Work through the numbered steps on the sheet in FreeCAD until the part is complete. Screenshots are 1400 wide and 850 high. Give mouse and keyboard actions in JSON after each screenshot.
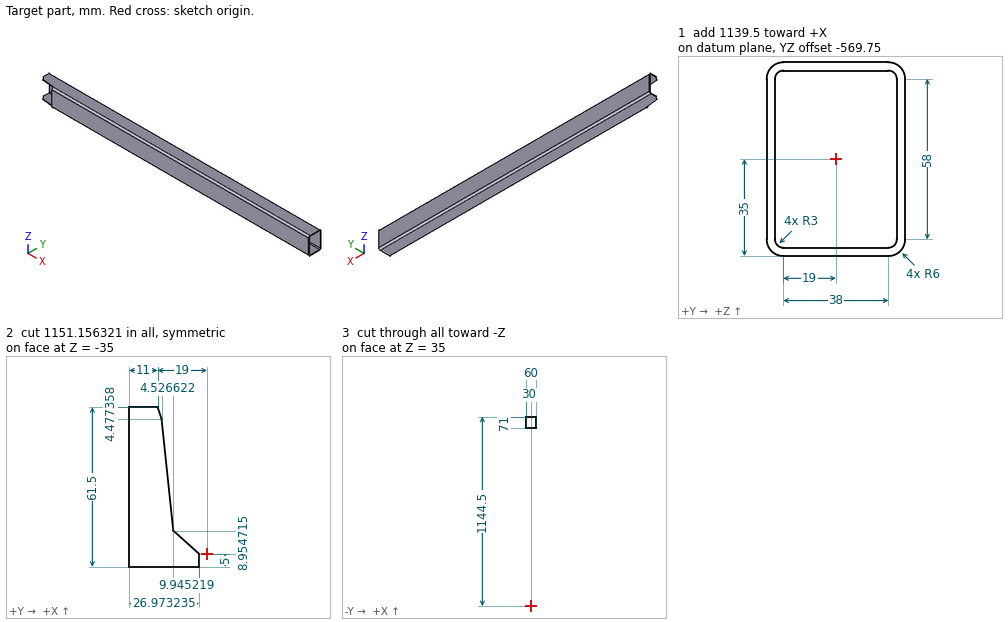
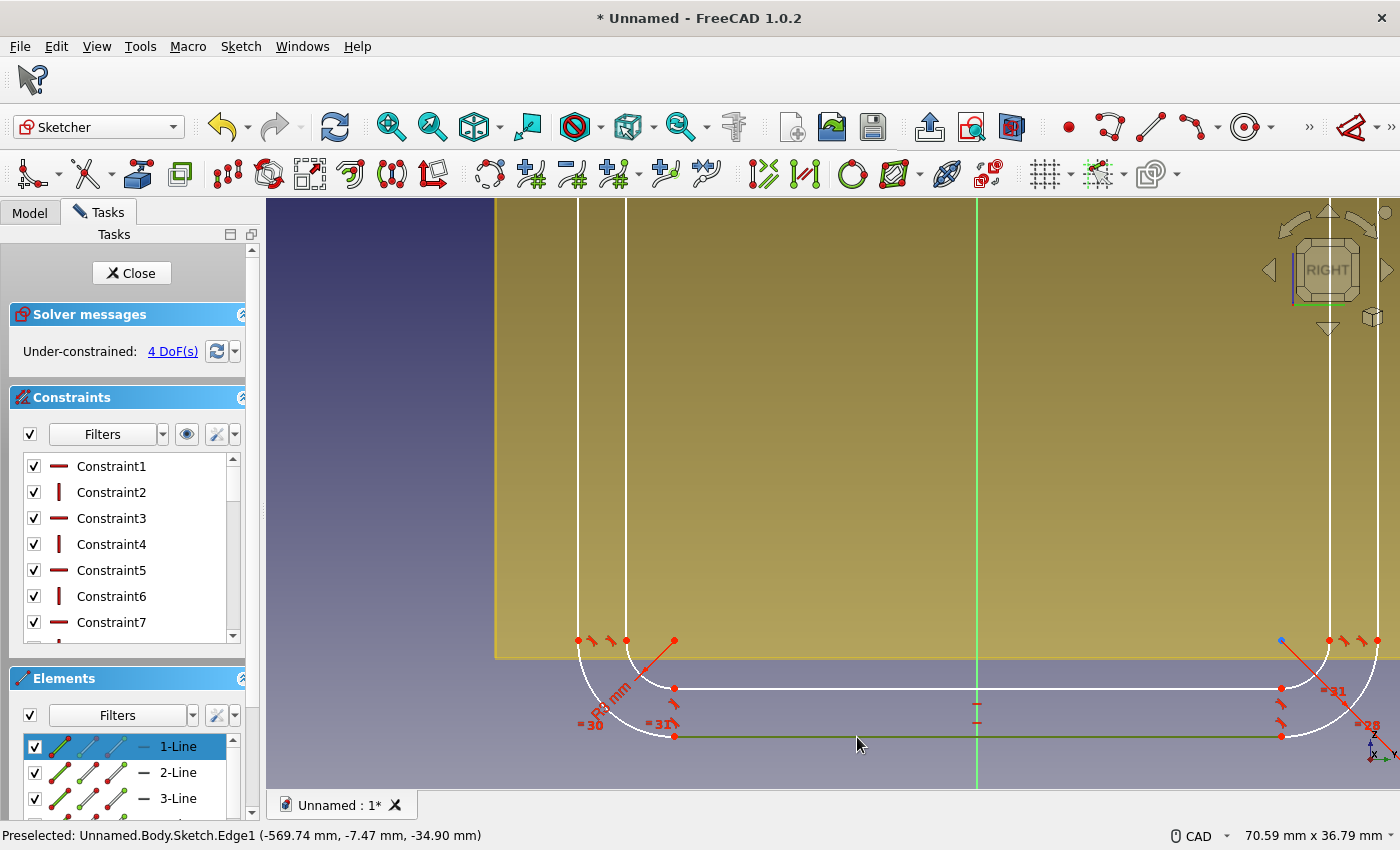
{"action": "key", "text": "l"}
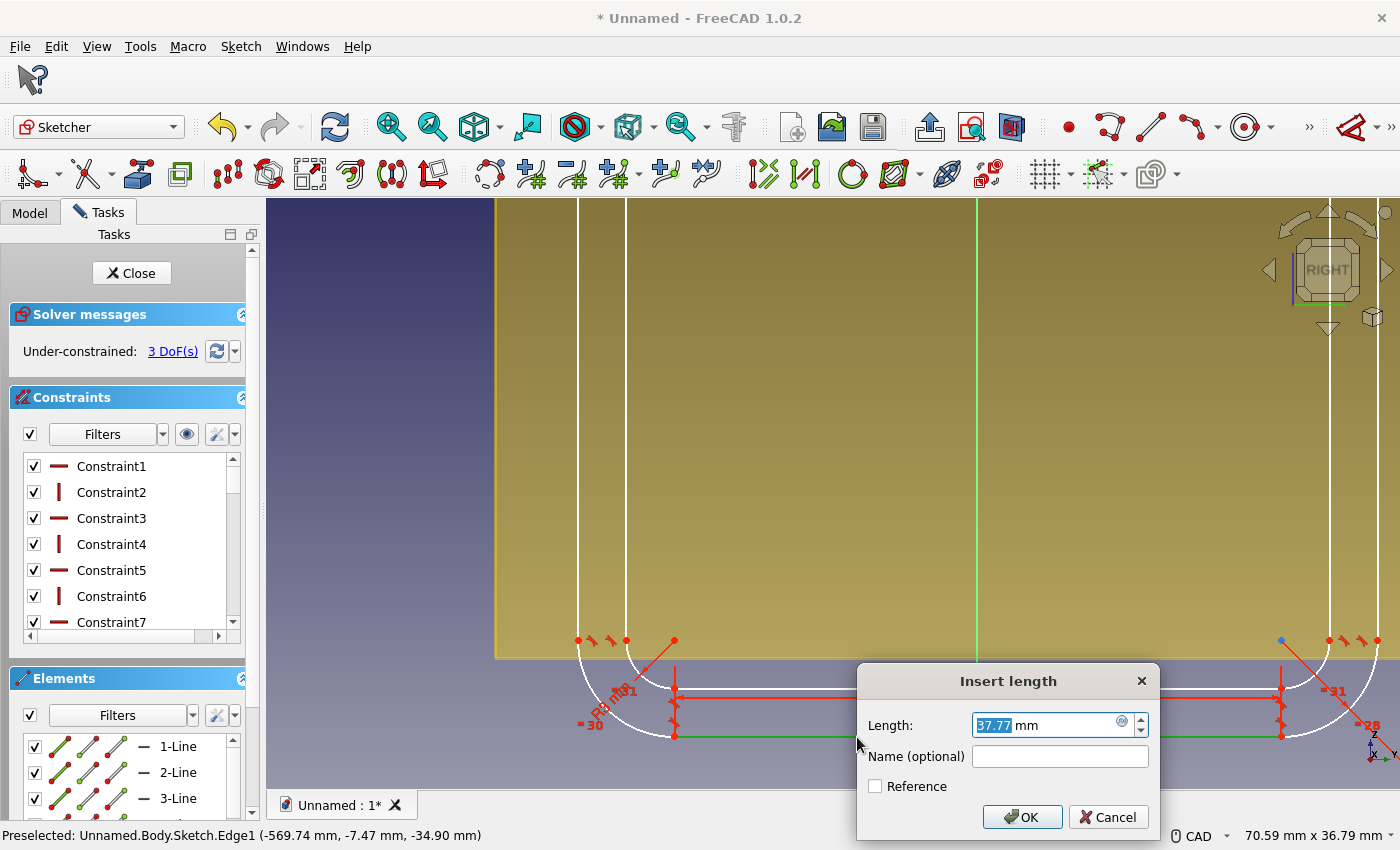
{"action": "type", "text": "38"}
{"action": "key", "text": "Return"}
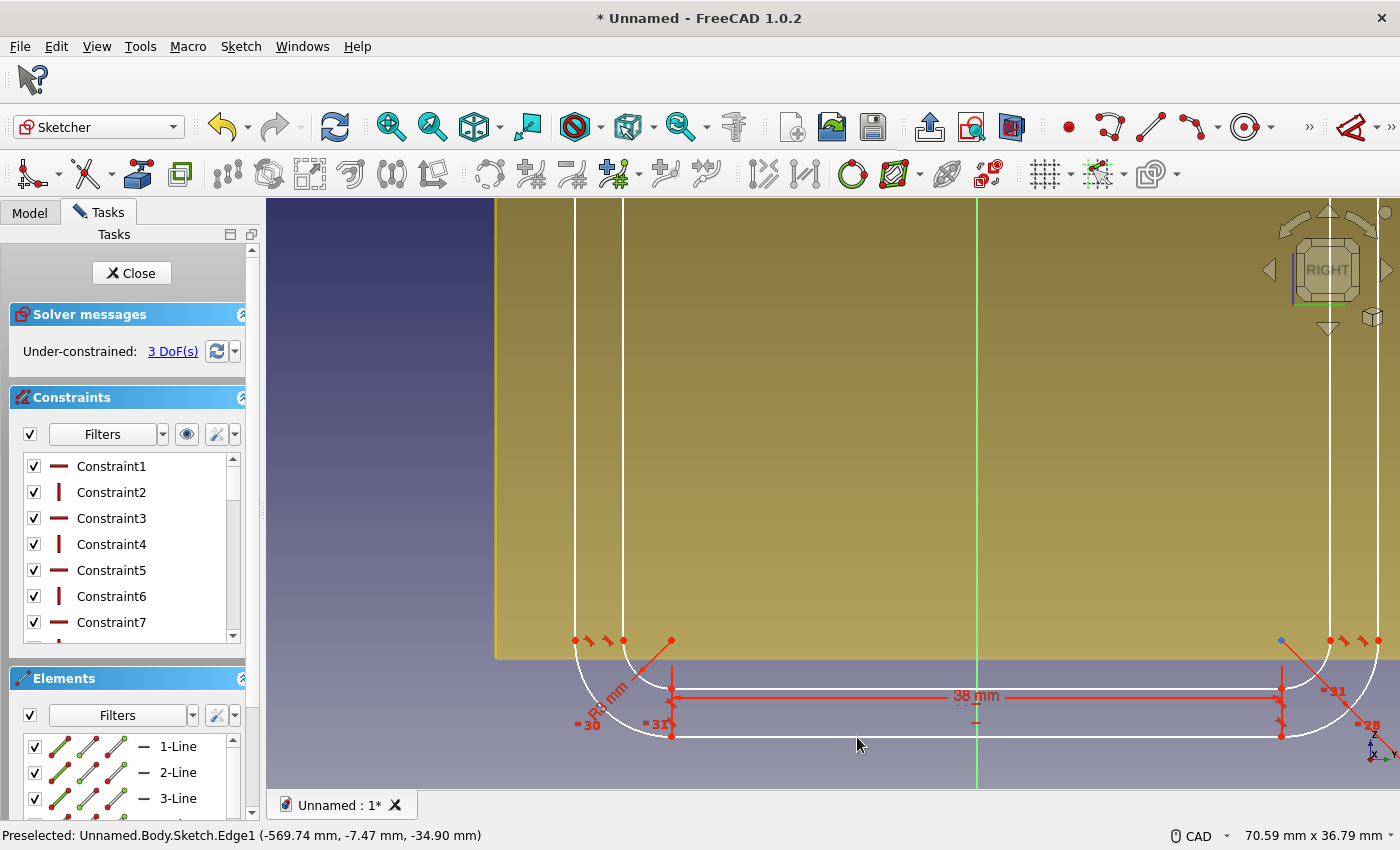
{"action": "scroll", "coordinate": [641, 678], "scroll_direction": "down", "scroll_amount": 5}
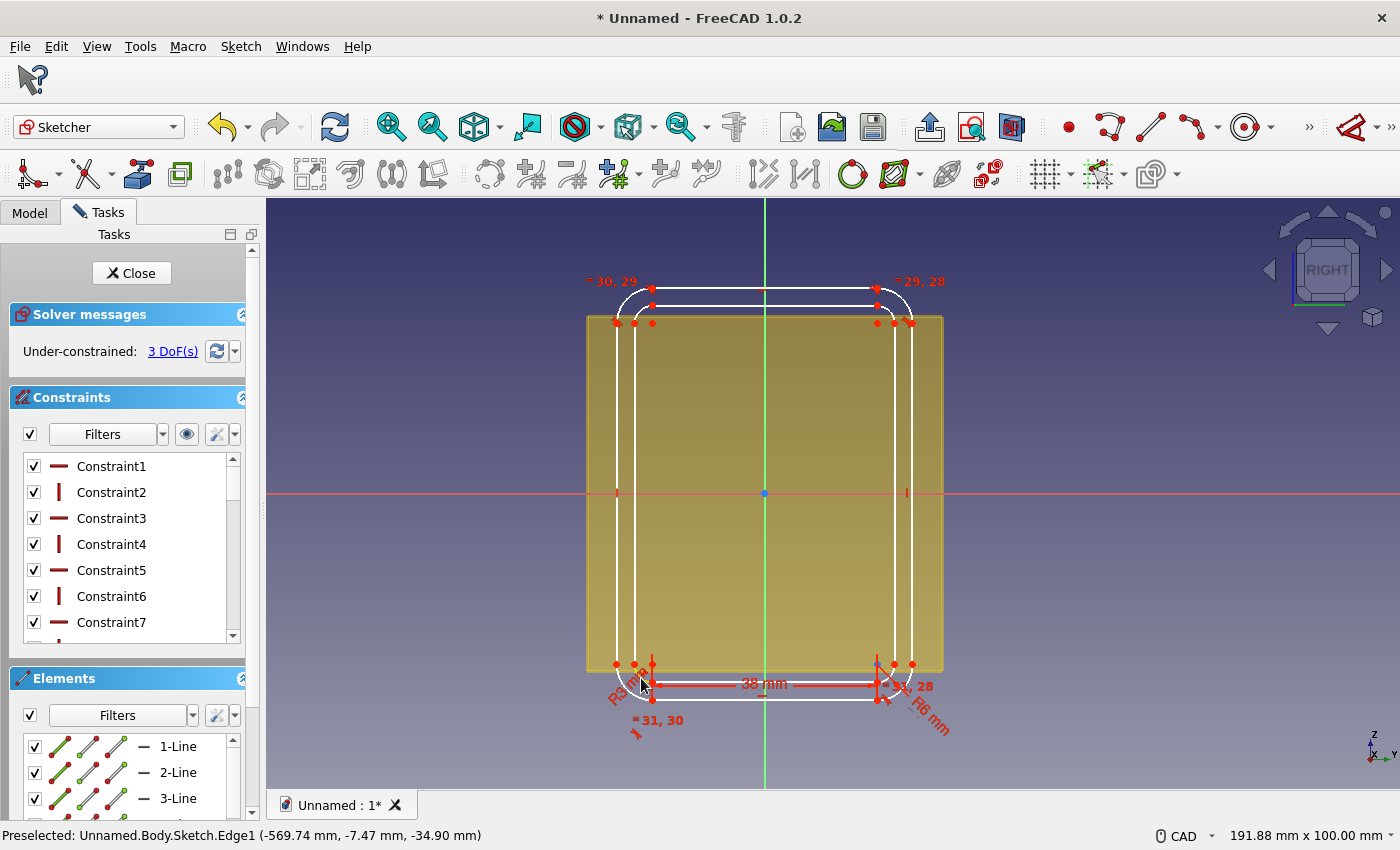
{"action": "left_click", "coordinate": [912, 562]}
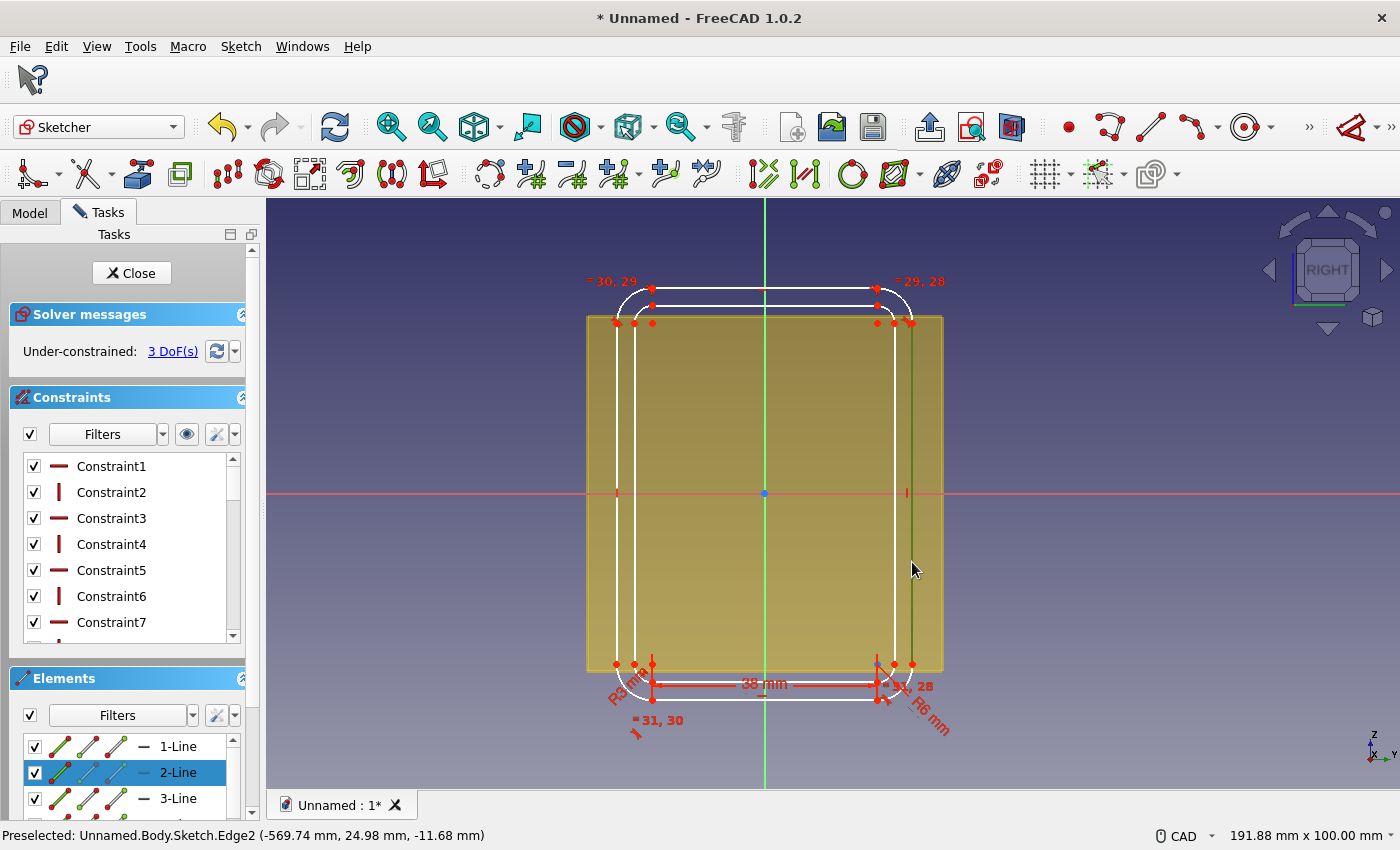
{"action": "key", "text": "i"}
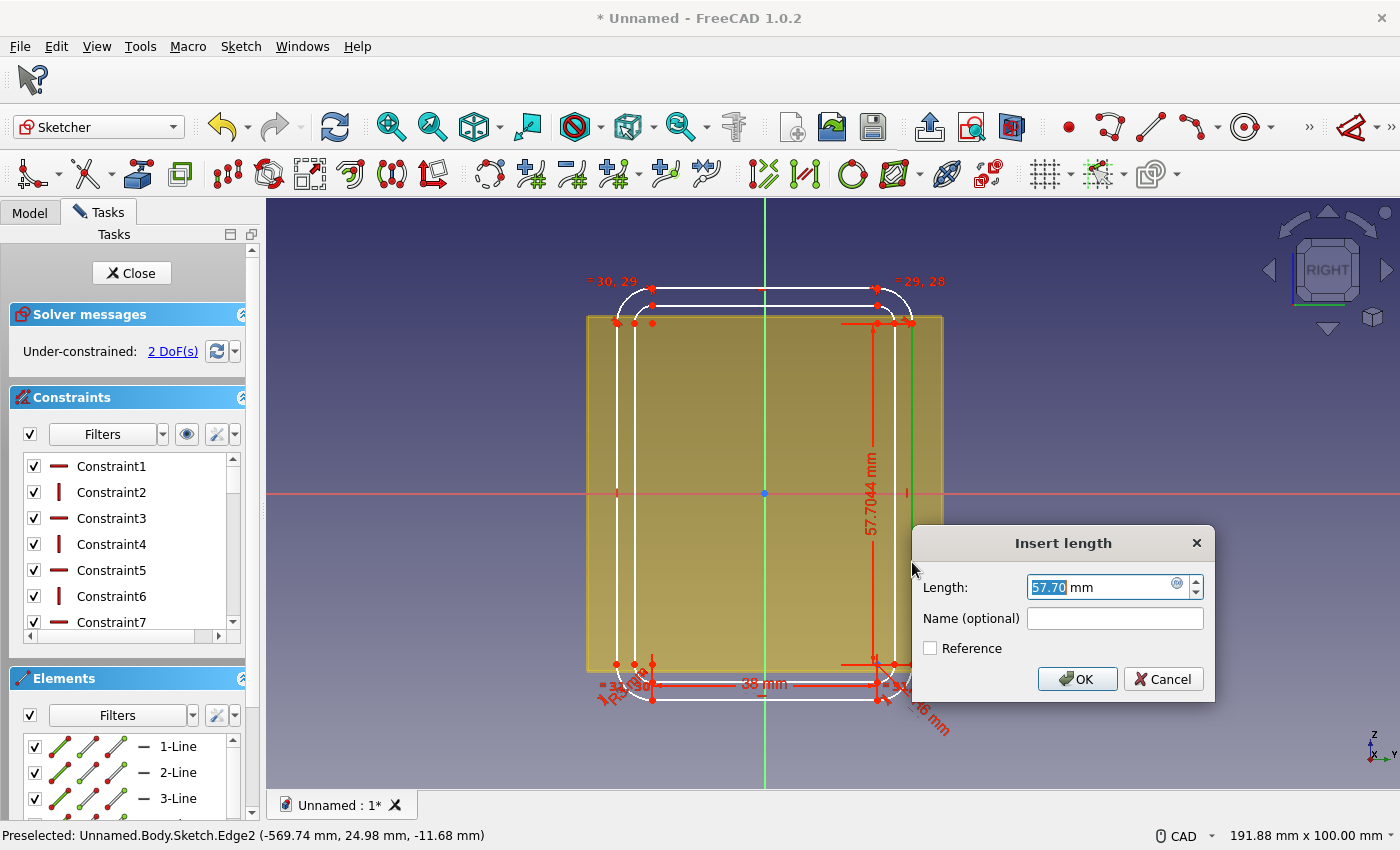
{"action": "type", "text": "58"}
{"action": "key", "text": "Return"}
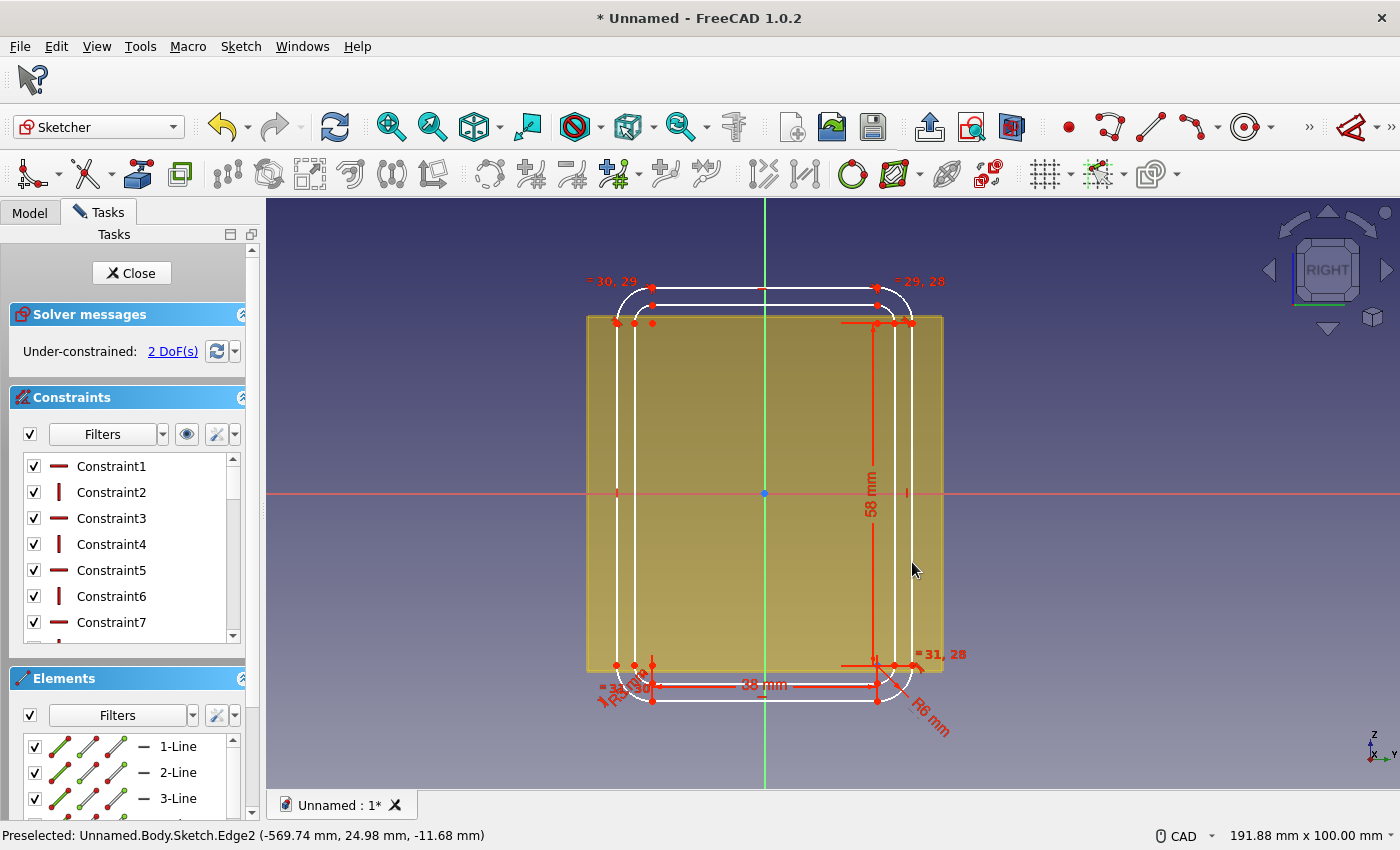
{"action": "left_click", "coordinate": [652, 701]}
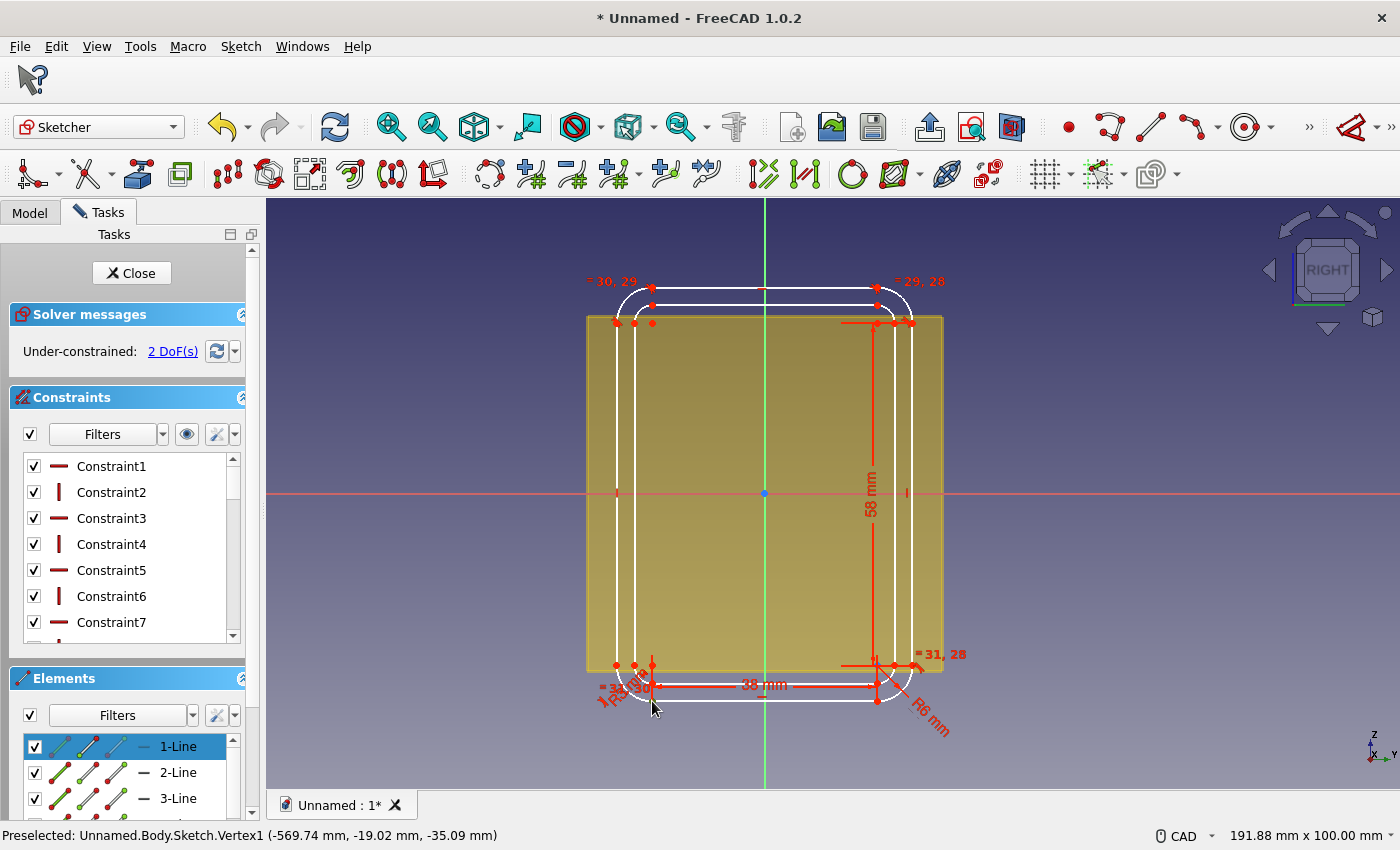
{"action": "key", "text": "l"}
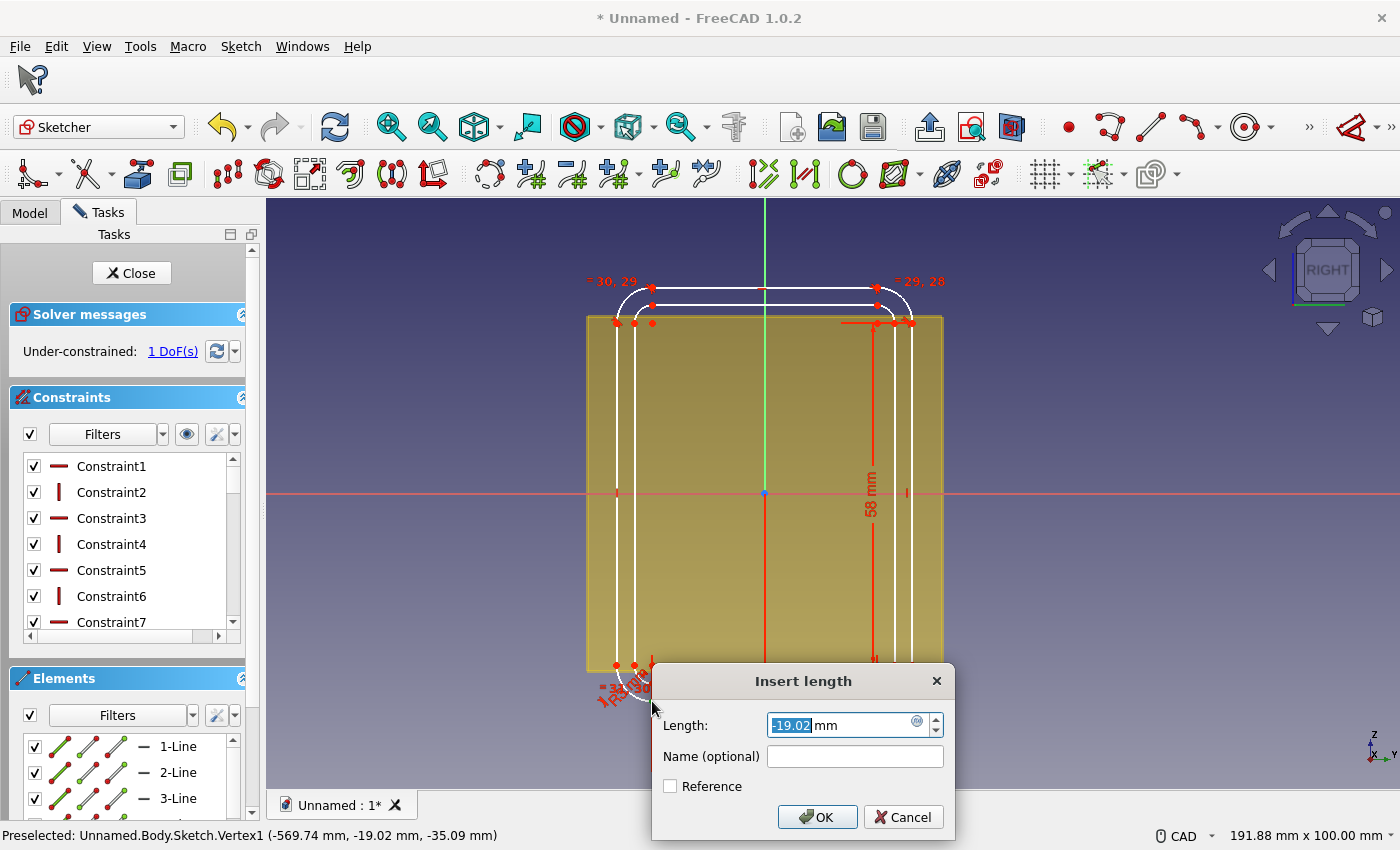
{"action": "type", "text": "-19"}
{"action": "key", "text": "Return"}